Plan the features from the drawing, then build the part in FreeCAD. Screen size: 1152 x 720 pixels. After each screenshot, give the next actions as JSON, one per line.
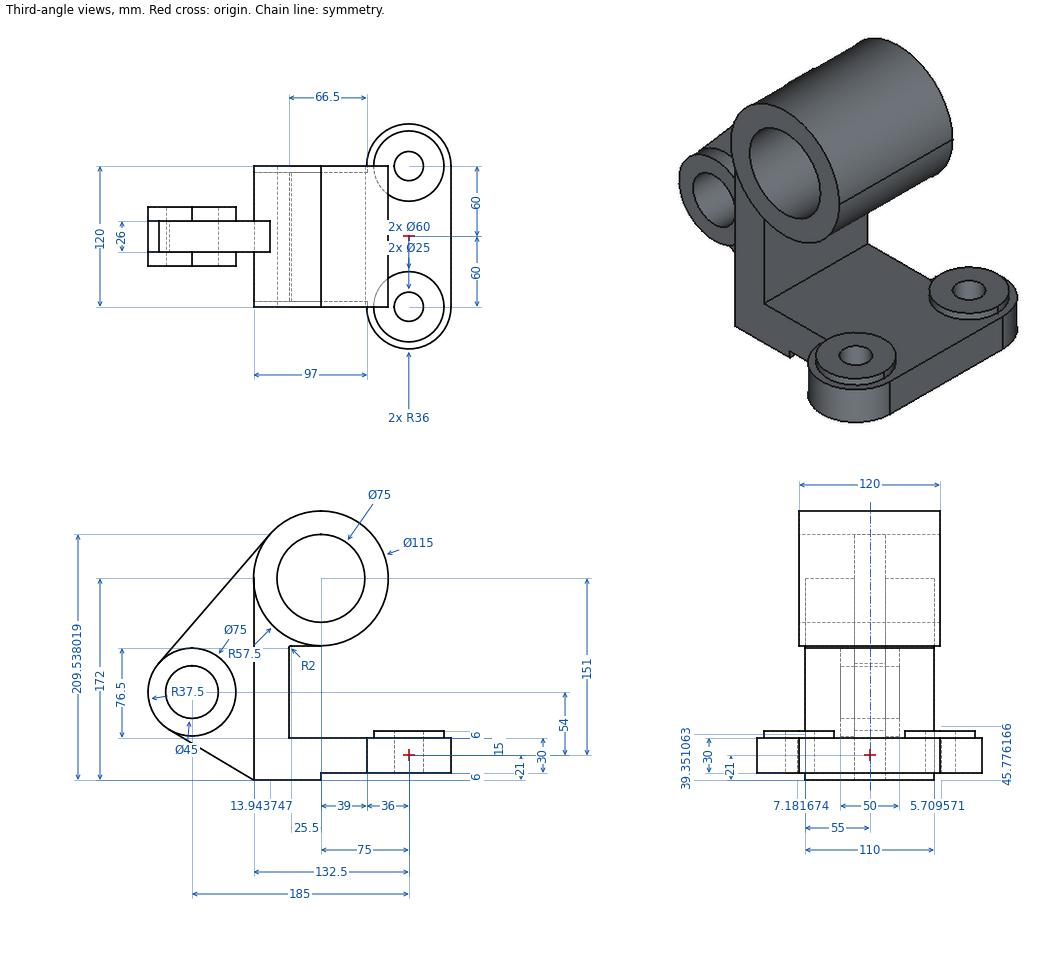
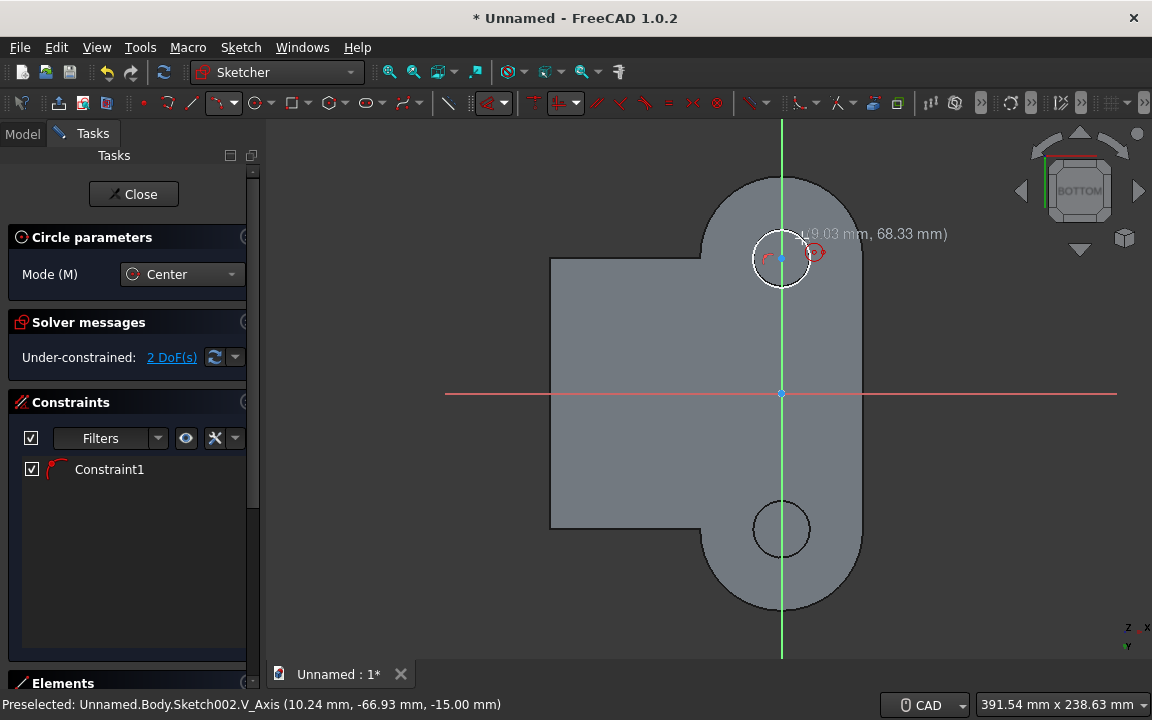
{"action": "left_click", "coordinate": [782, 529]}
{"action": "left_click", "coordinate": [802, 509]}
{"action": "key", "text": "Escape"}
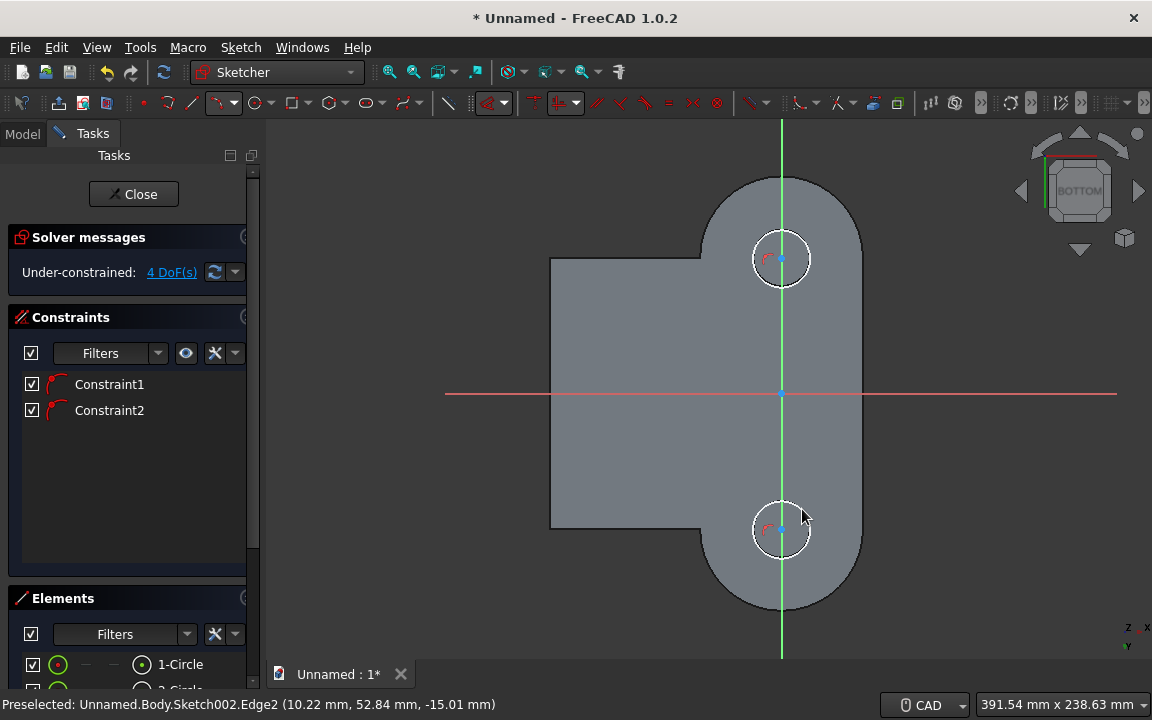
{"action": "left_click", "coordinate": [802, 239]}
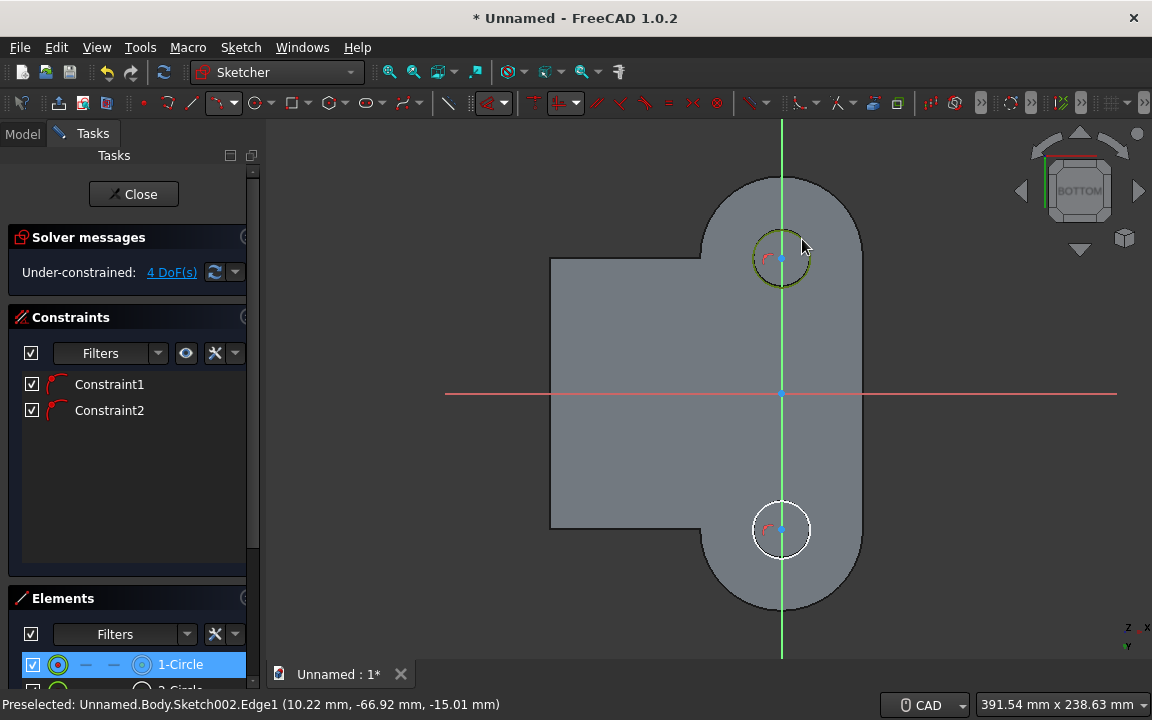
{"action": "left_click", "coordinate": [802, 510]}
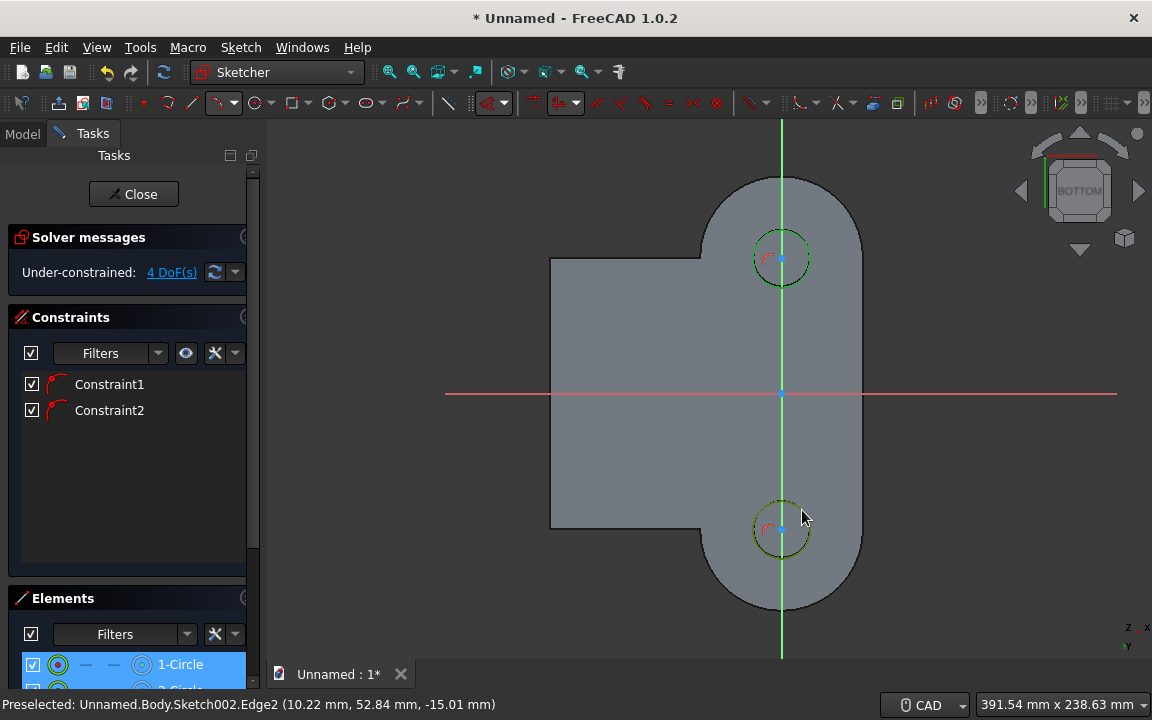
{"action": "left_click", "coordinate": [670, 104]}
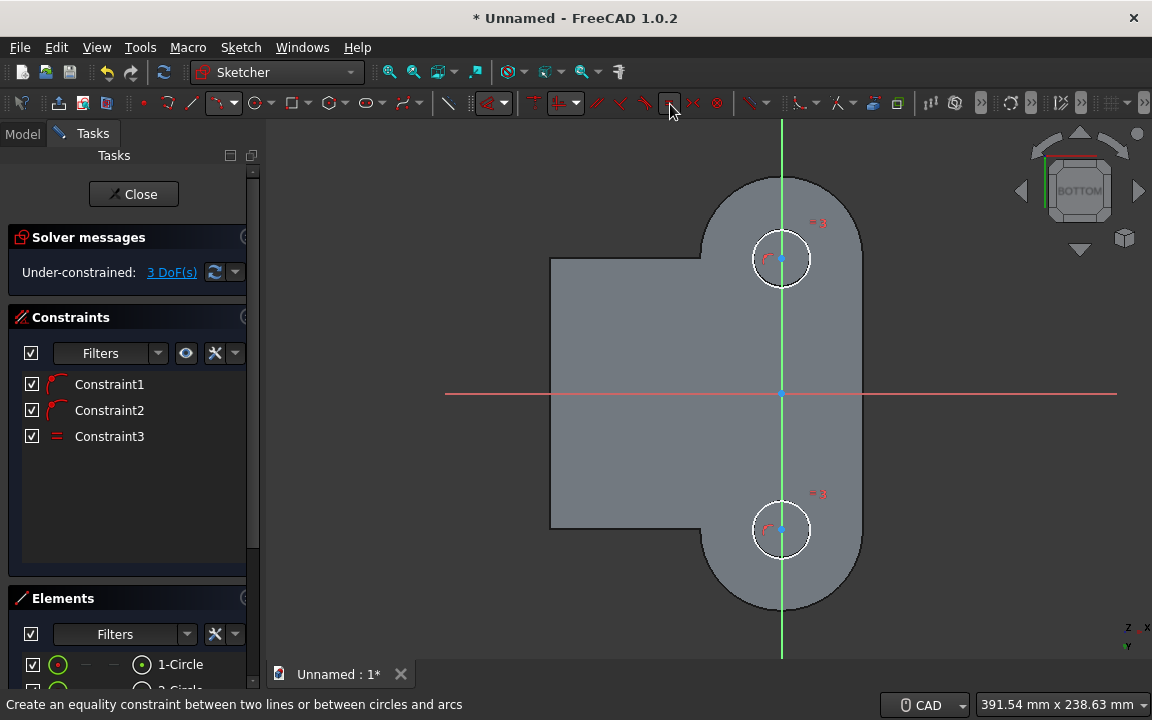
{"action": "left_click", "coordinate": [802, 239]}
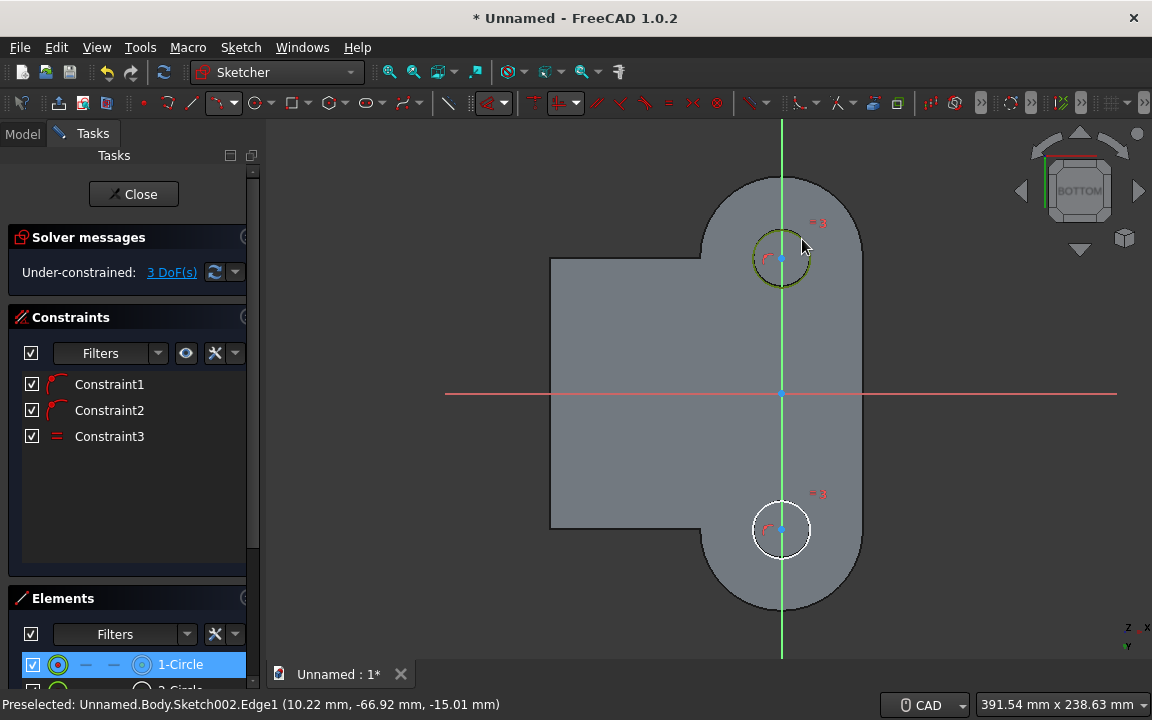
{"action": "key", "text": "k o"}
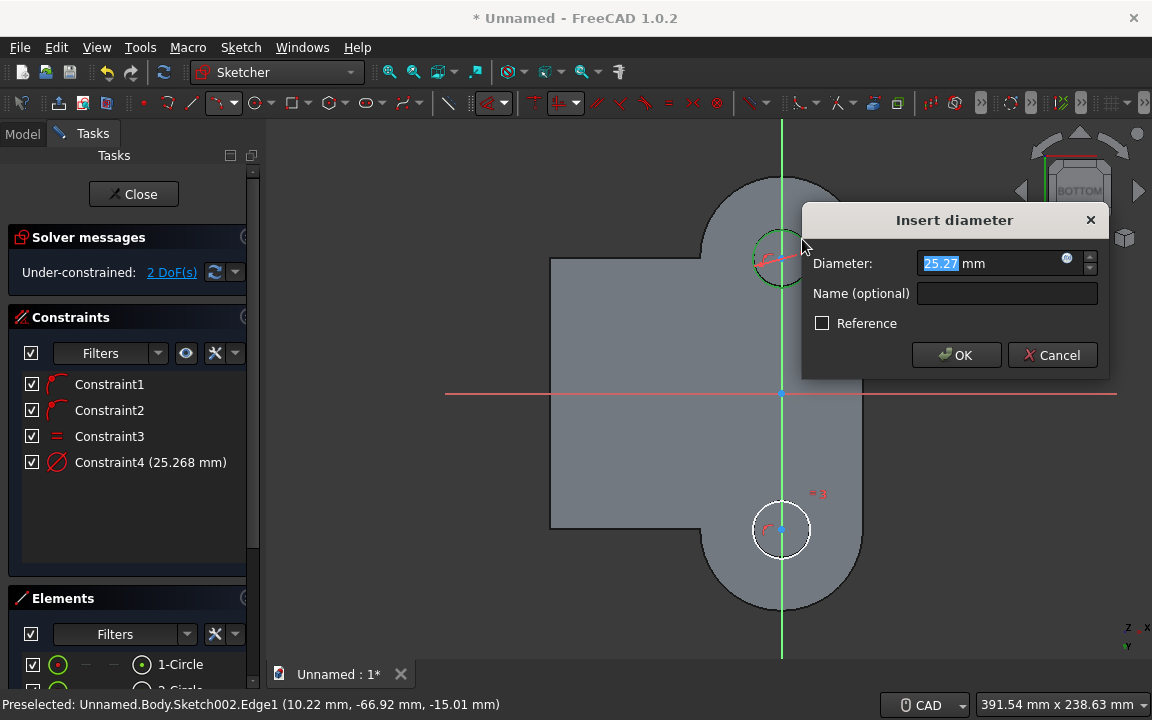
{"action": "type", "text": "25"}
{"action": "key", "text": "Return"}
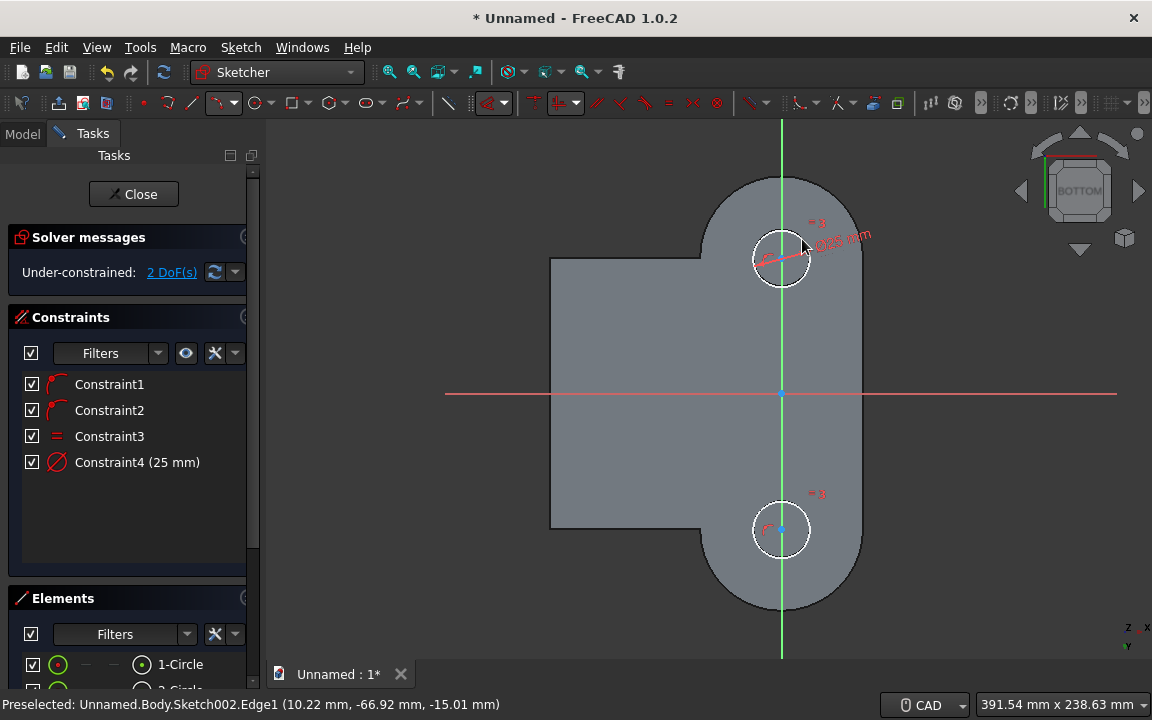
{"action": "left_click", "coordinate": [782, 259]}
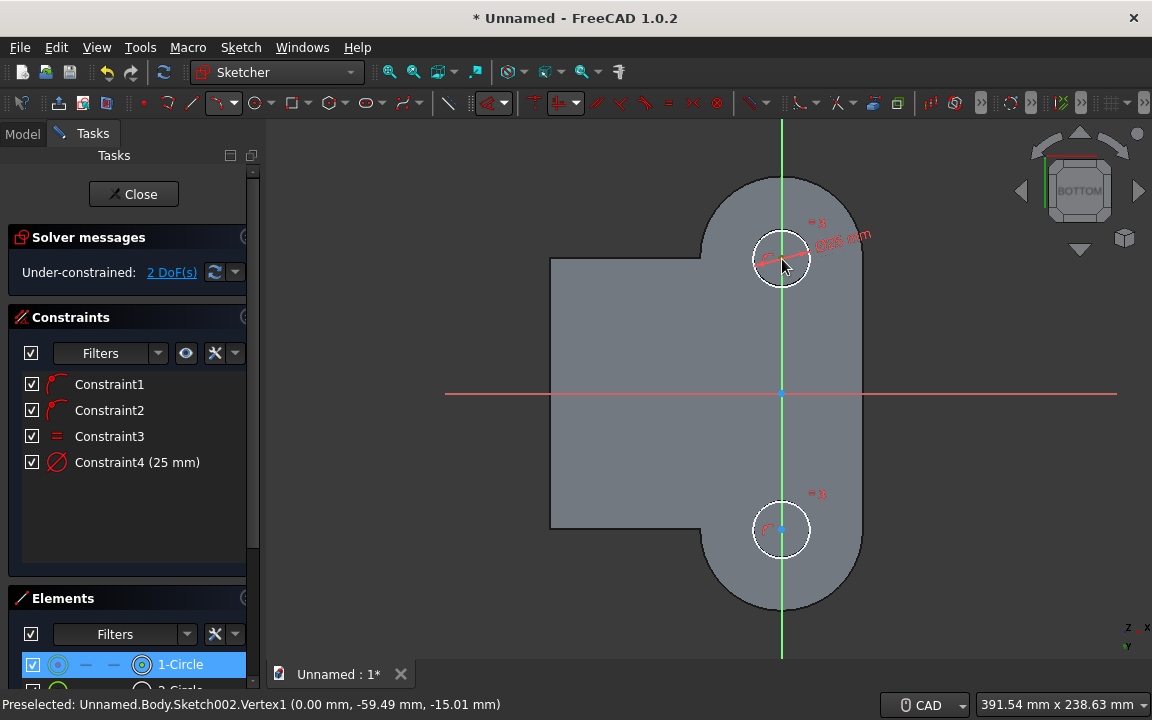
{"action": "key", "text": "i"}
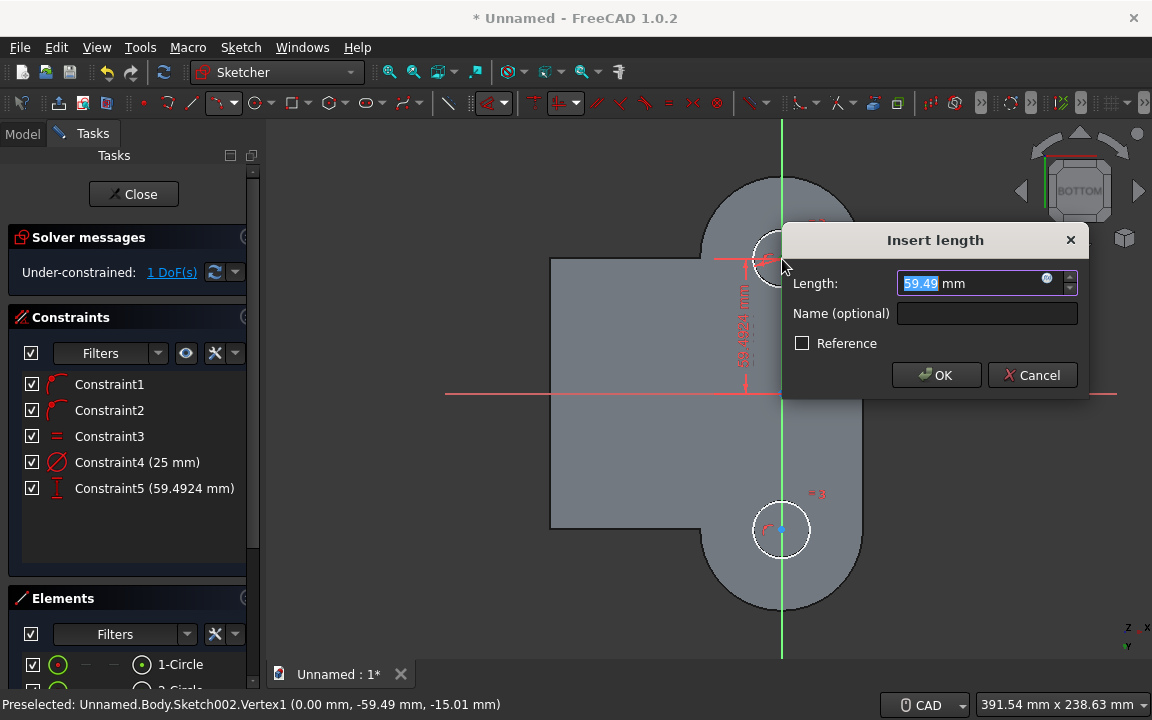
{"action": "type", "text": "60"}
{"action": "key", "text": "Return"}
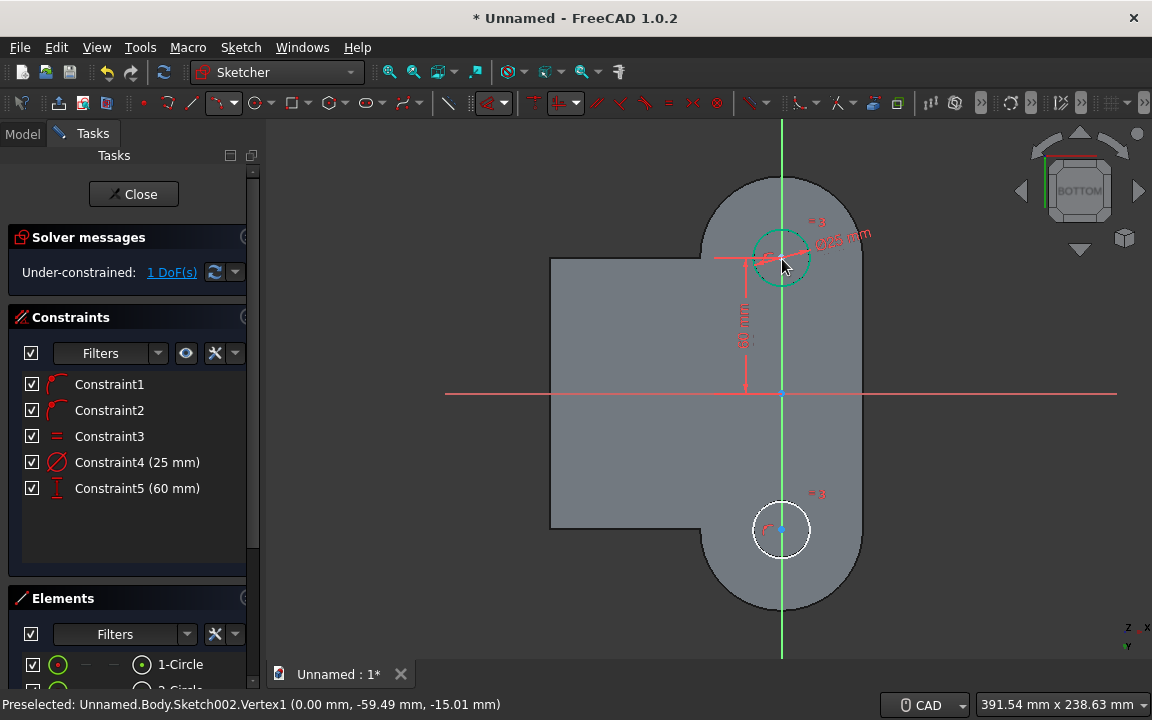
{"action": "left_click", "coordinate": [782, 530]}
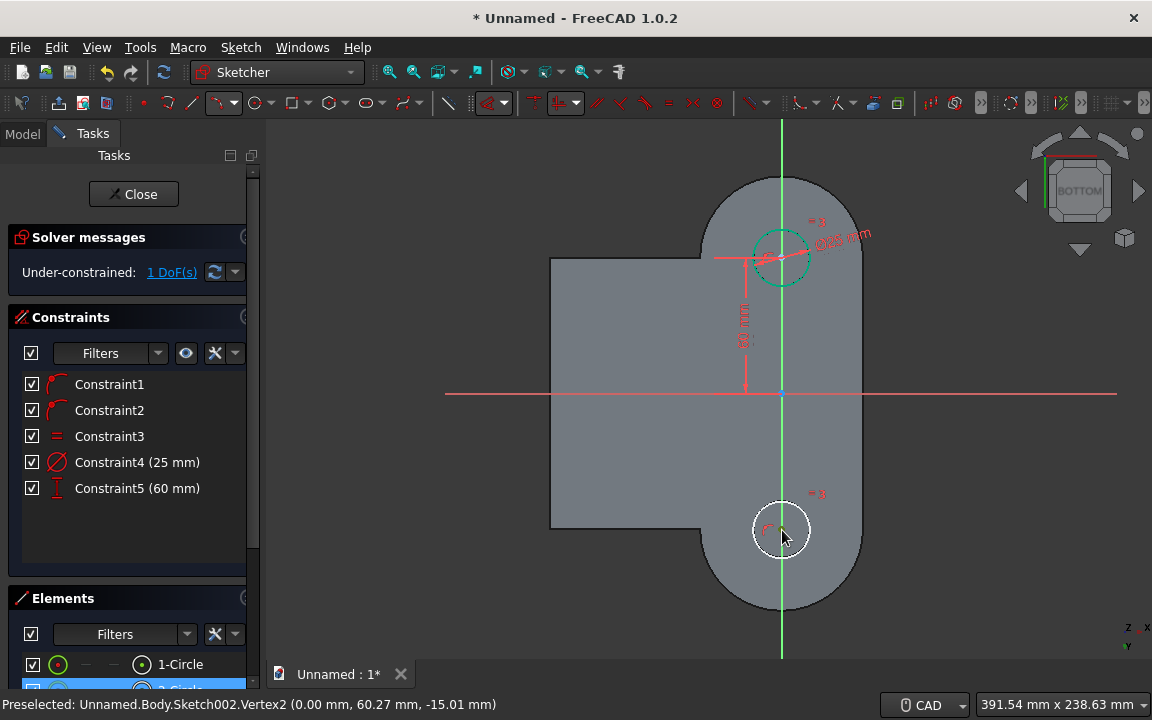
{"action": "key", "text": "i"}